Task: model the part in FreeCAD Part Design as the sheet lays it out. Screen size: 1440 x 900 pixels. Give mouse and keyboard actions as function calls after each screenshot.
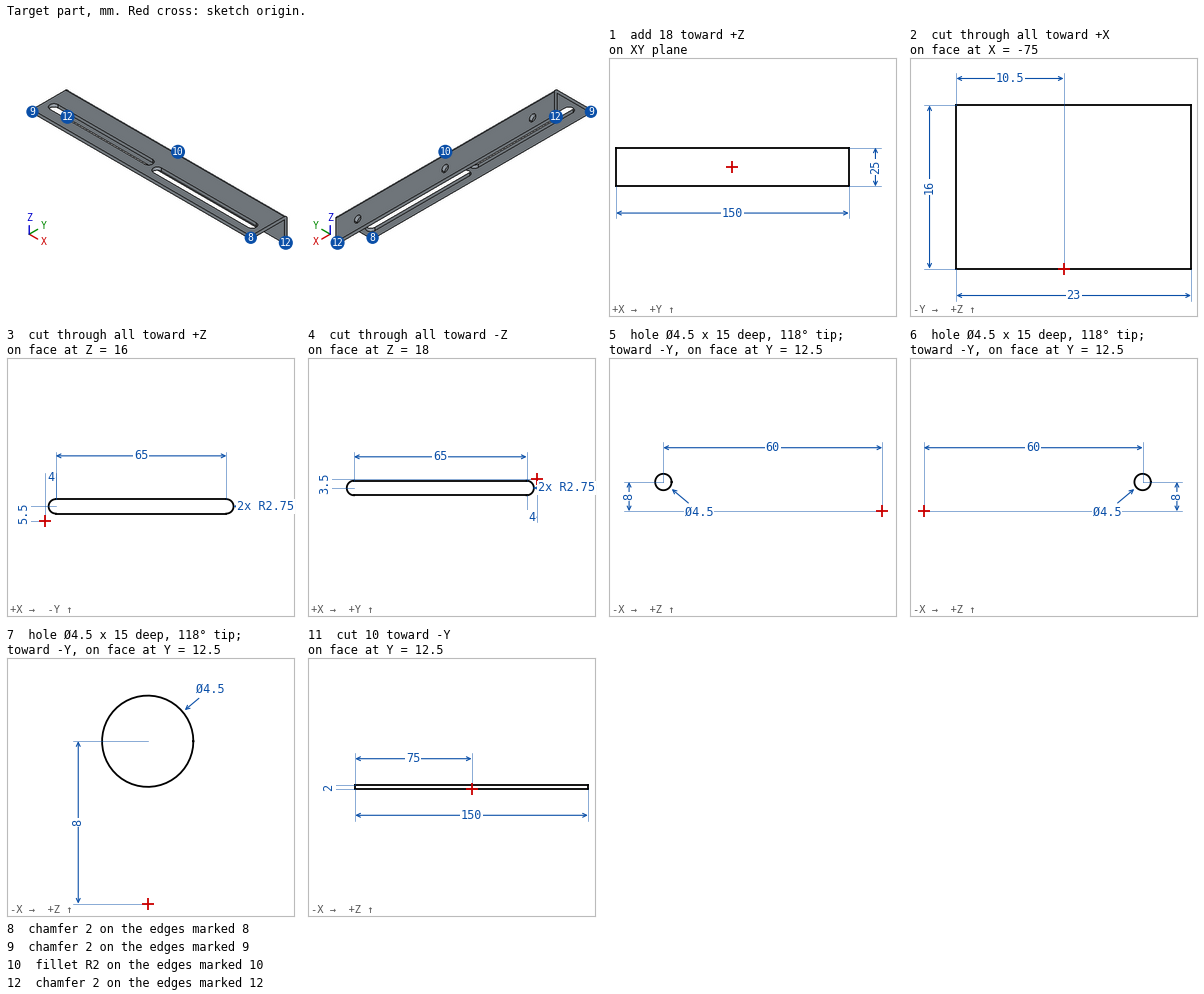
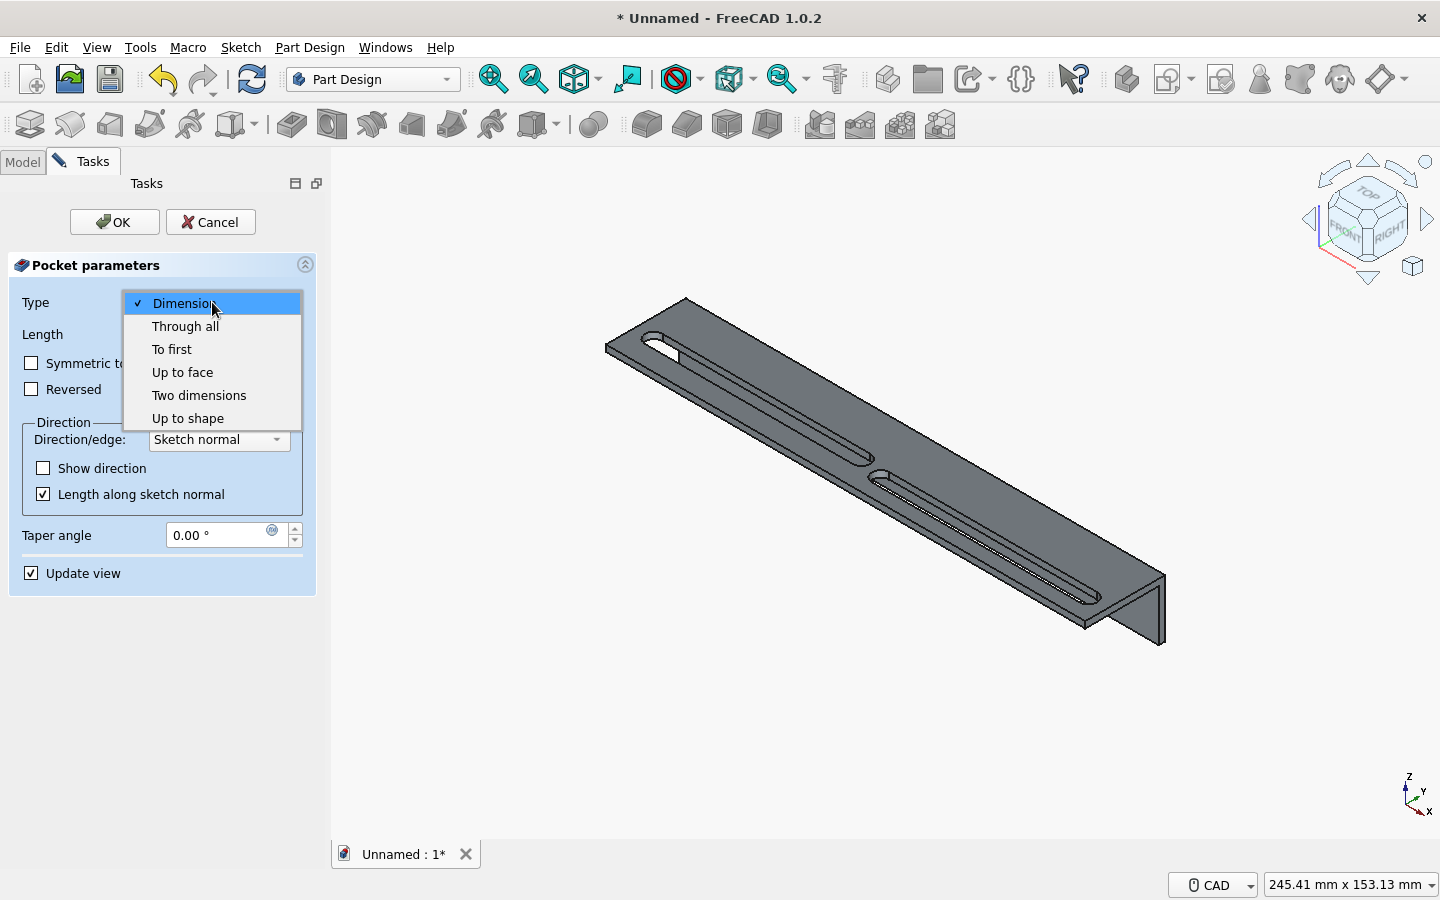
click(212, 326)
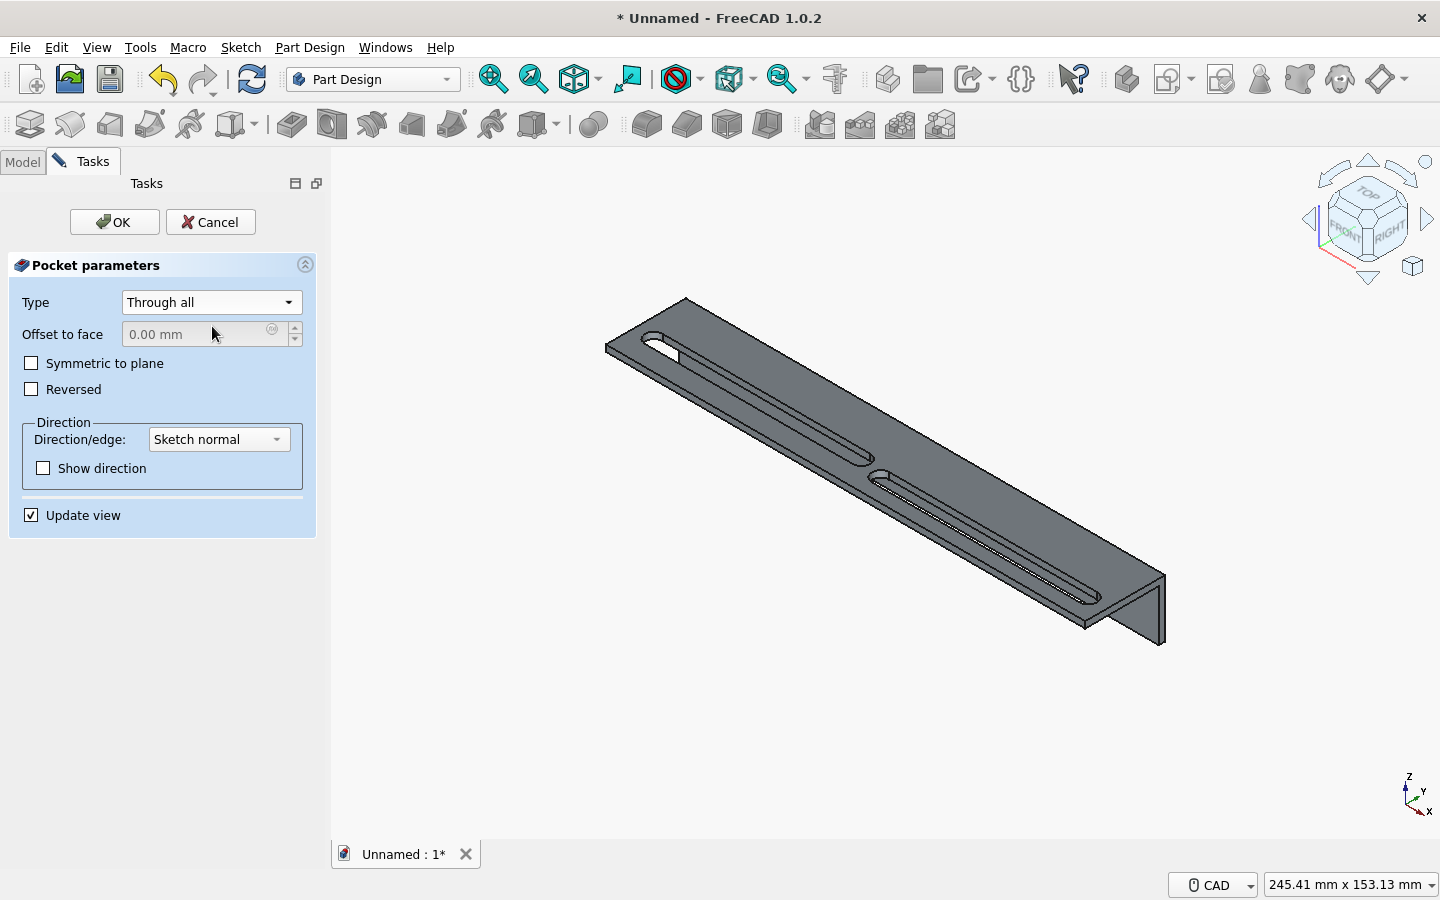
click(115, 222)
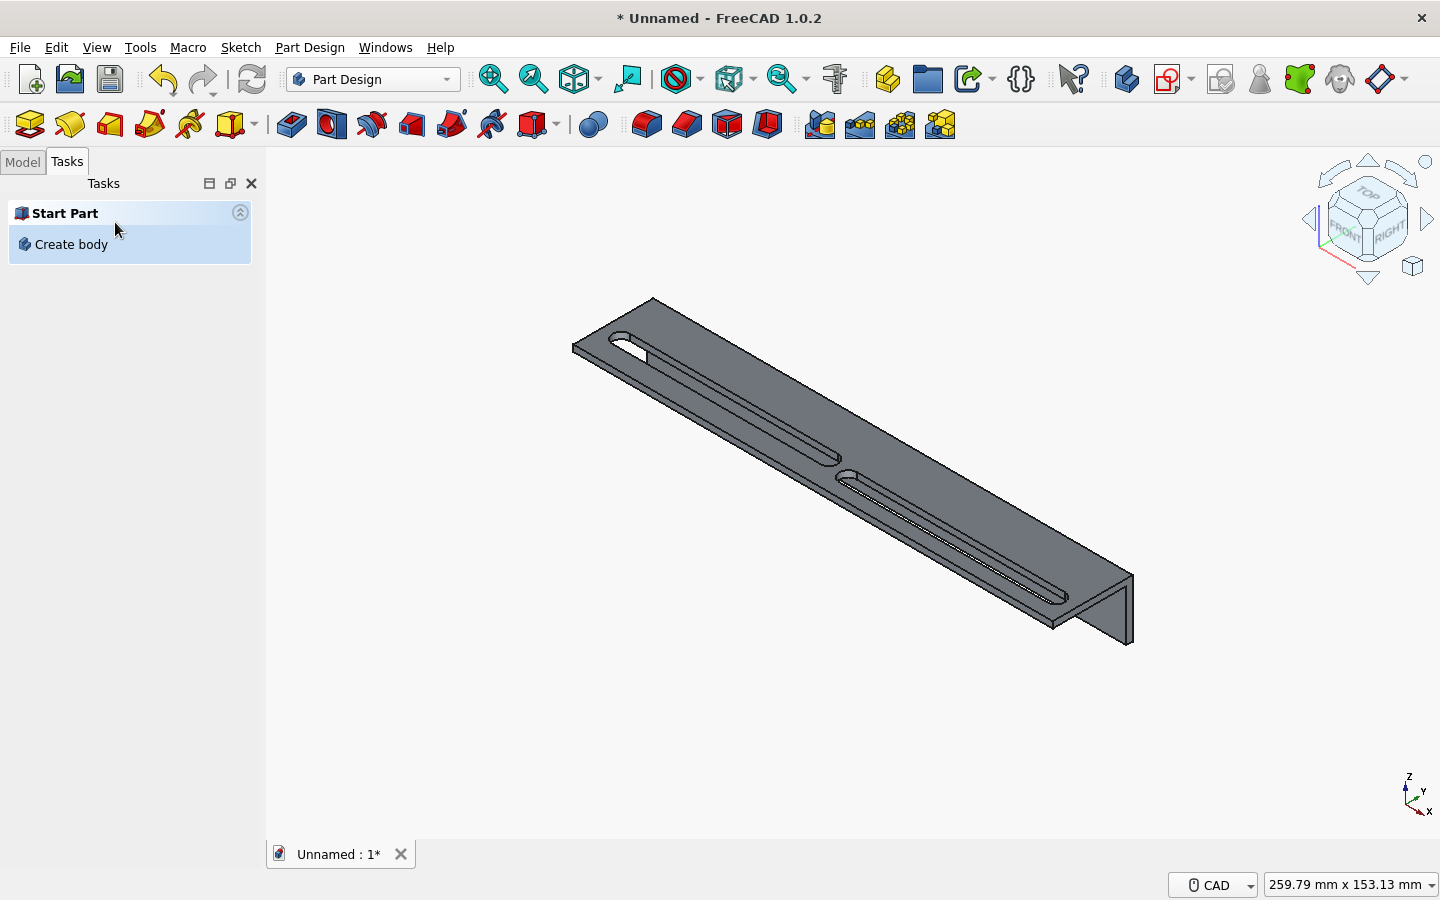
key(4)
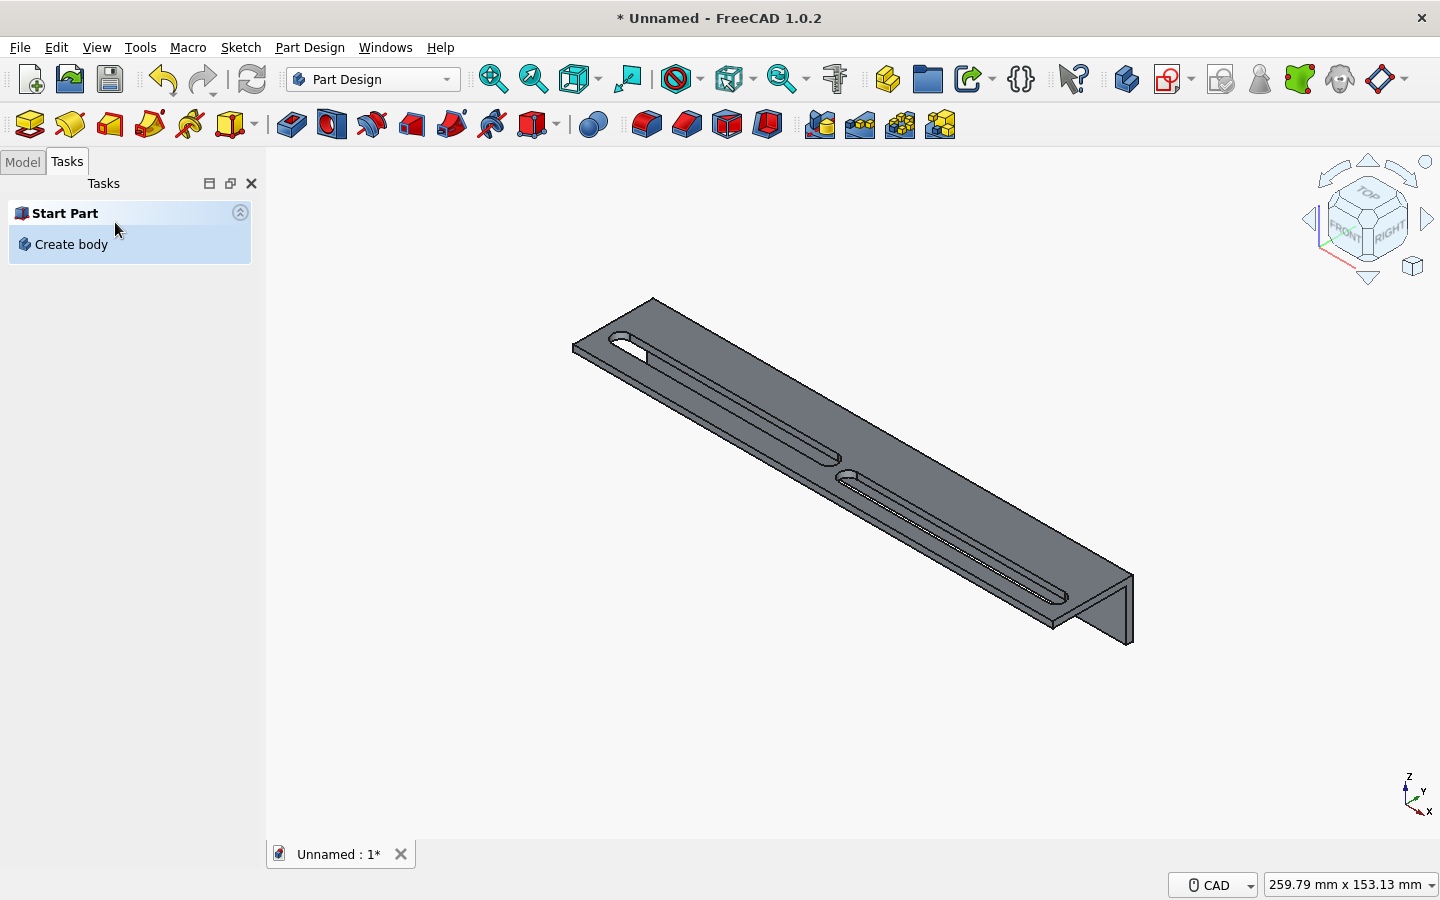
click(562, 492)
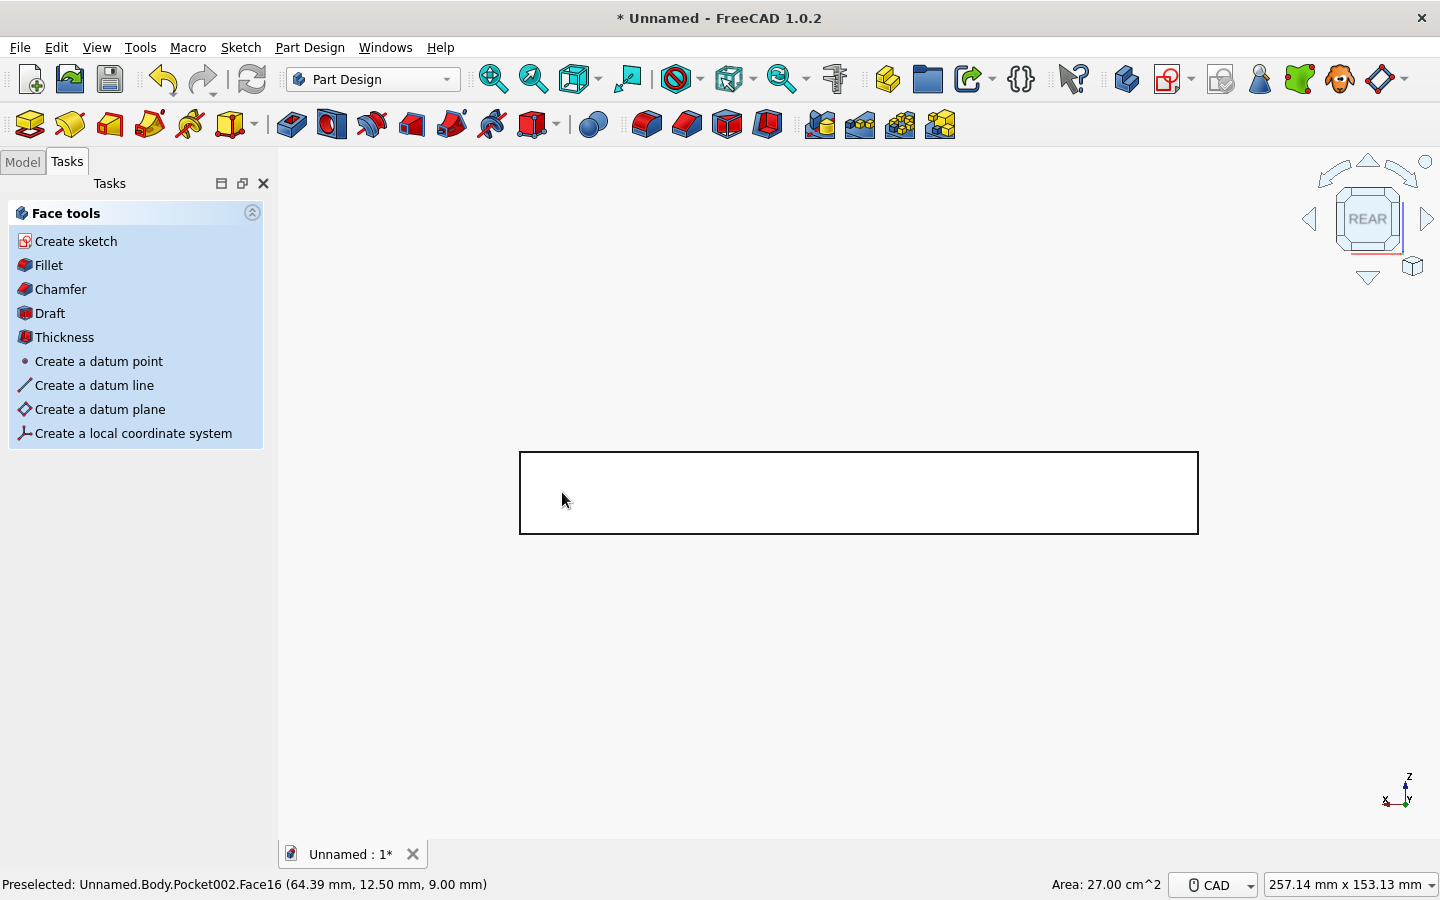
click(1168, 80)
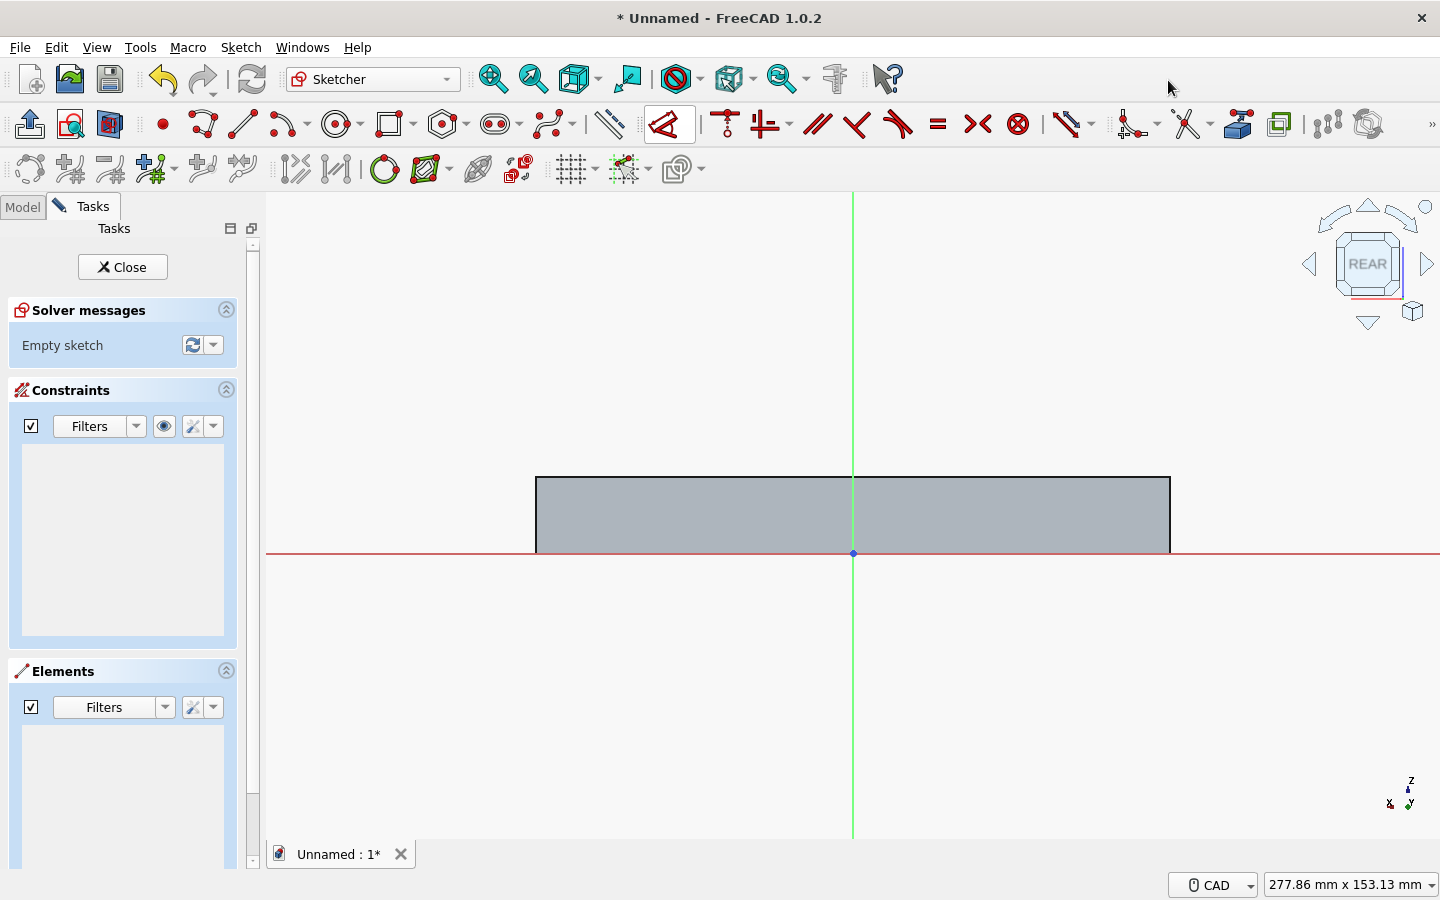
scroll(590, 520, up, 15)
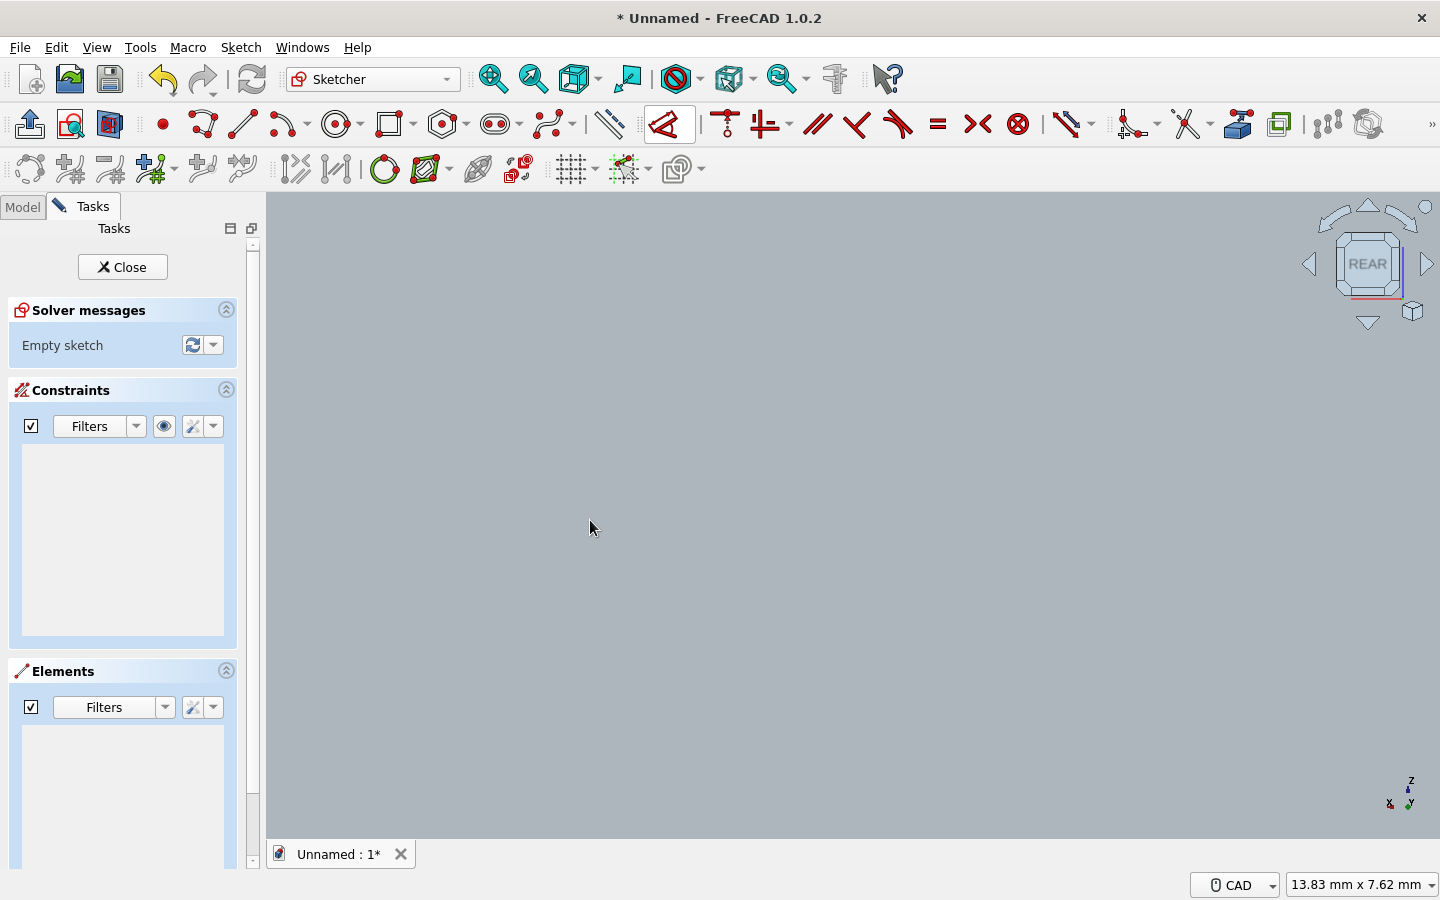
click(336, 124)